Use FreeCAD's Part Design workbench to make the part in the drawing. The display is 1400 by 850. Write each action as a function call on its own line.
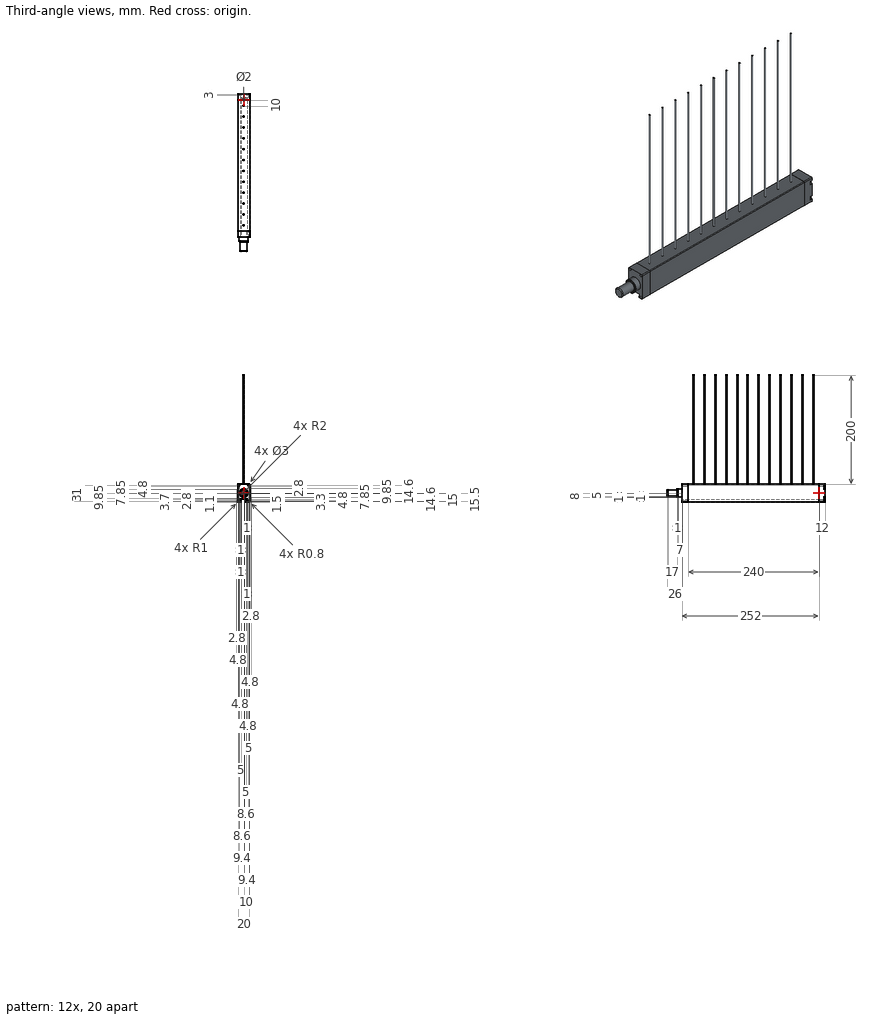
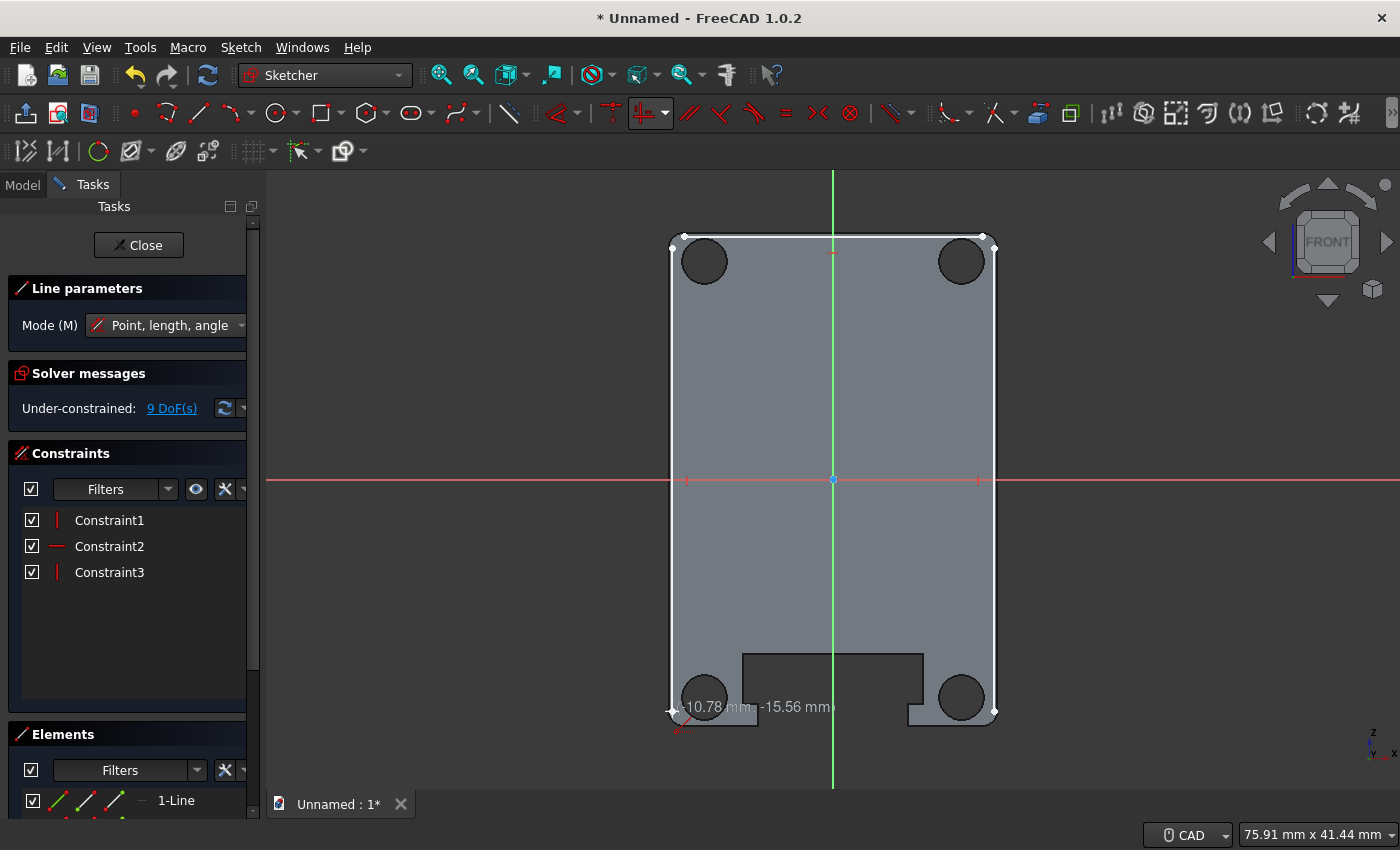
click(168, 114)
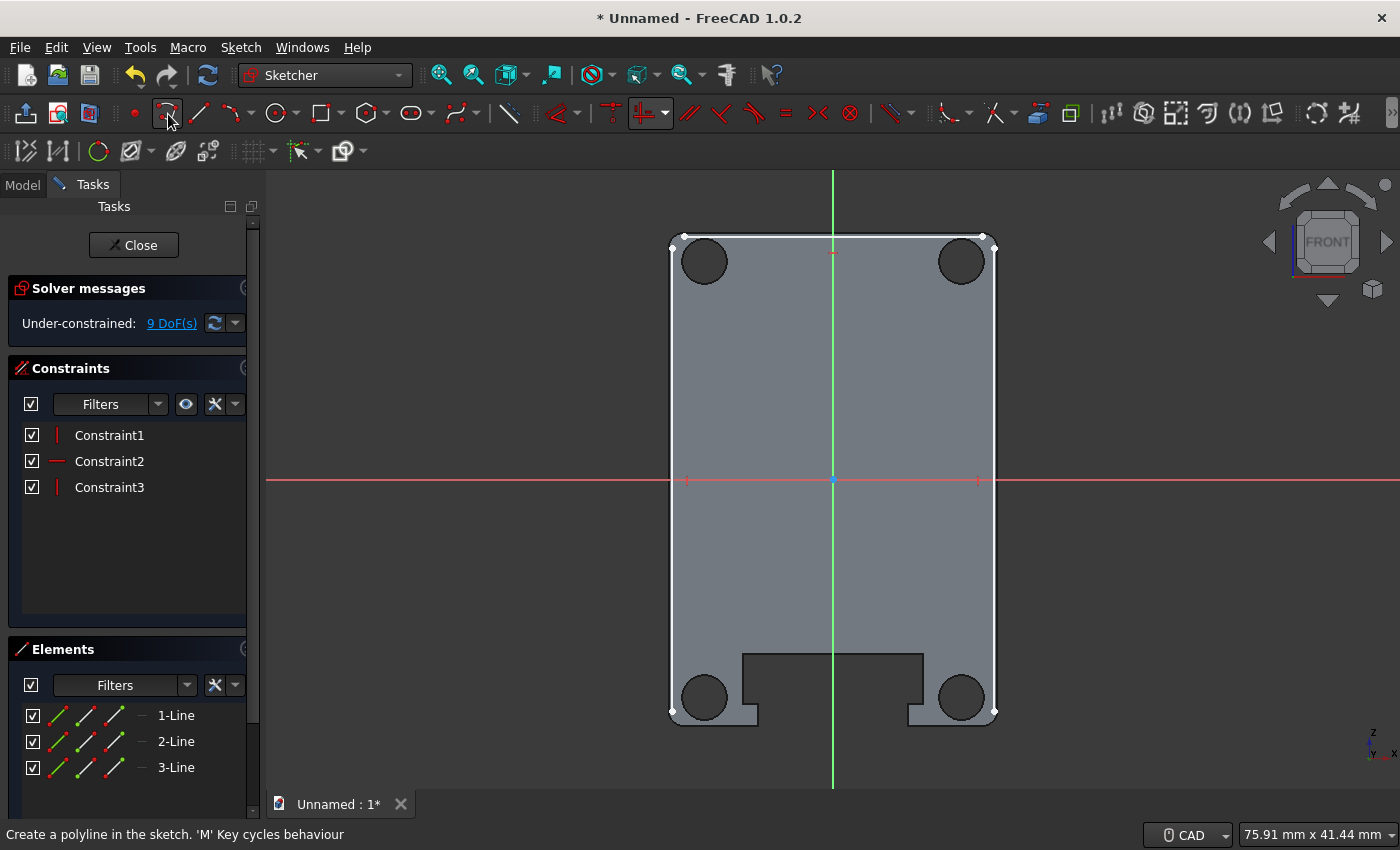
click(684, 723)
click(755, 723)
click(755, 707)
click(740, 707)
click(740, 651)
click(926, 651)
click(926, 707)
click(911, 707)
click(911, 723)
click(982, 723)
right_click(982, 723)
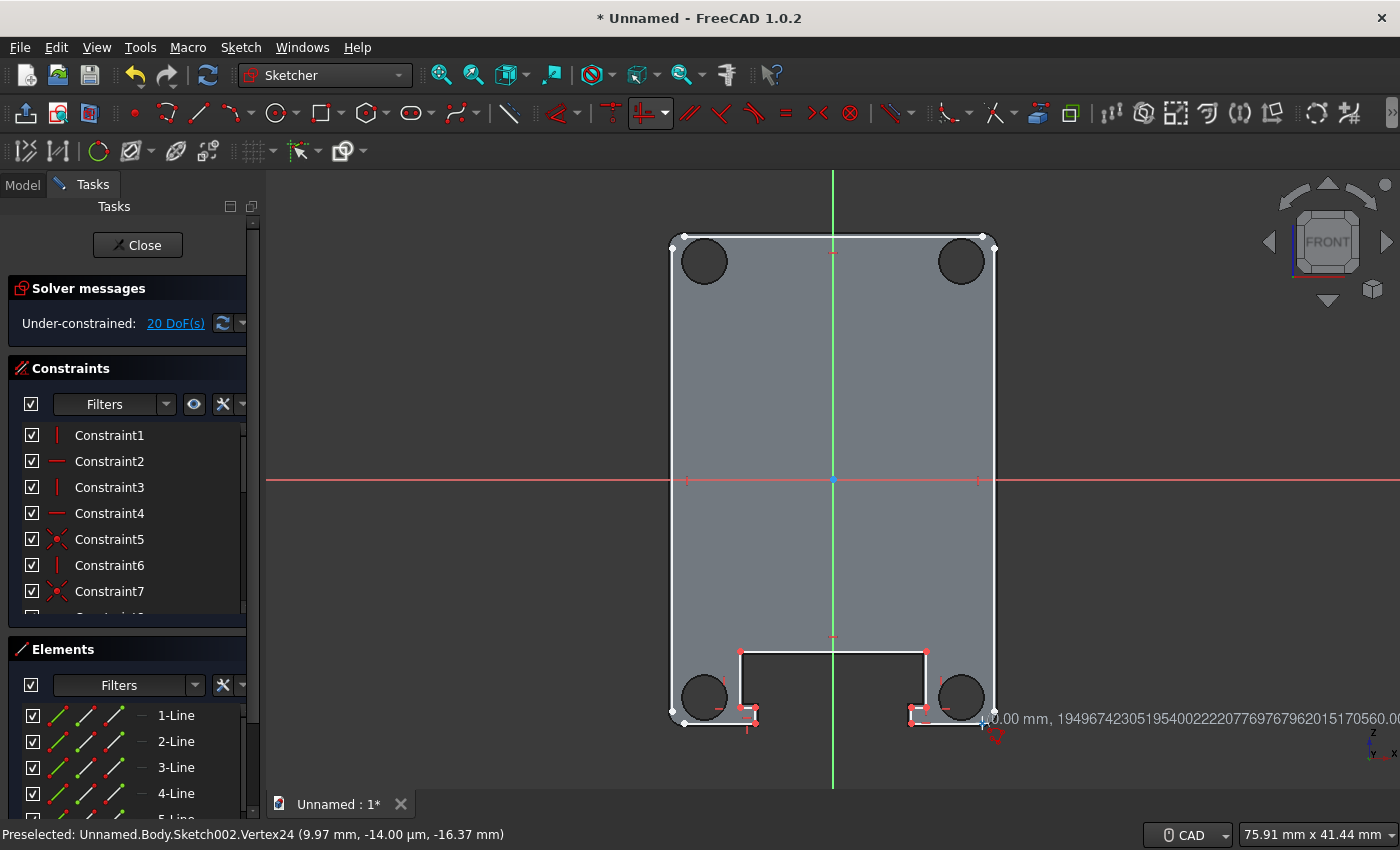
click(232, 114)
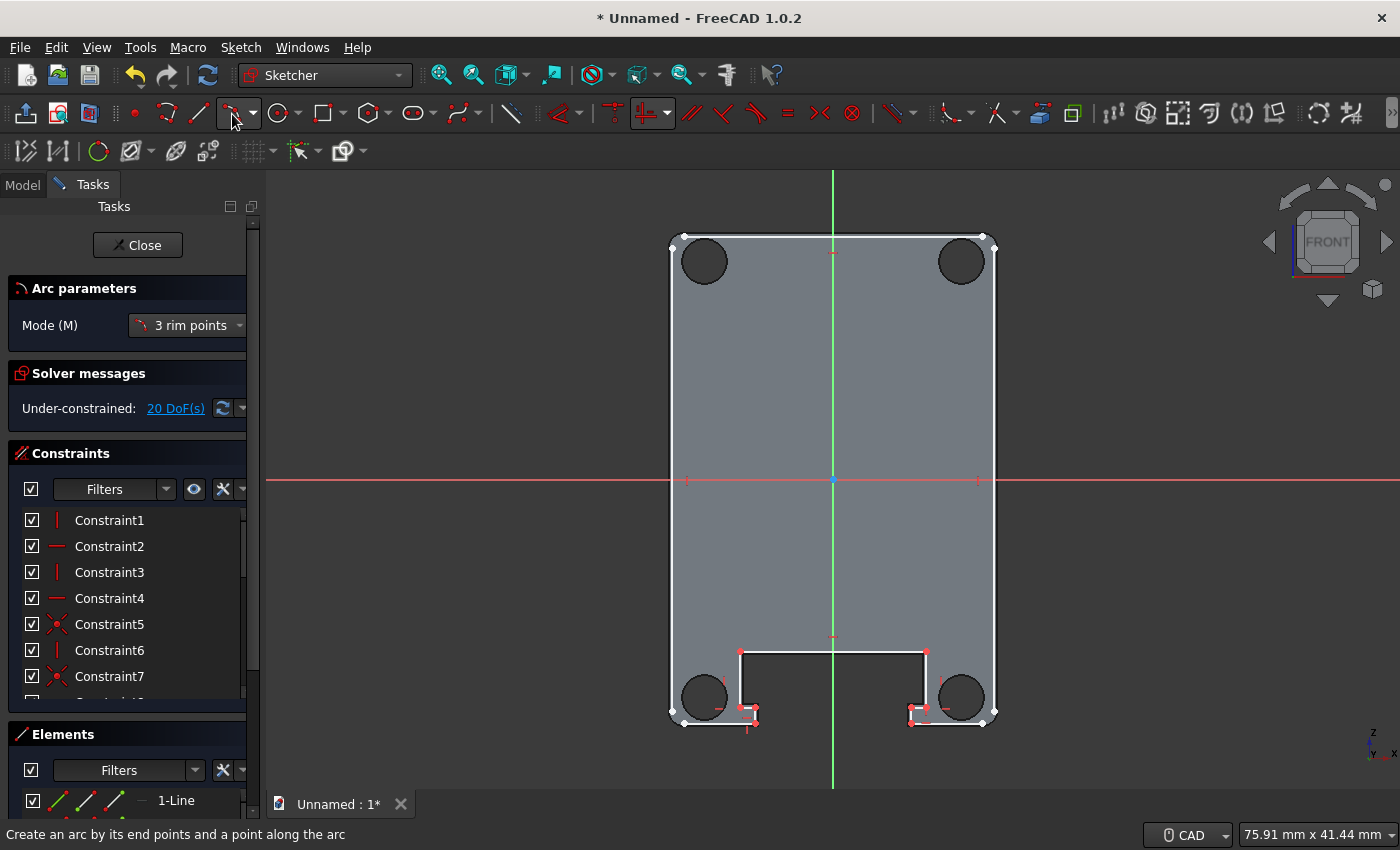
click(994, 249)
click(982, 237)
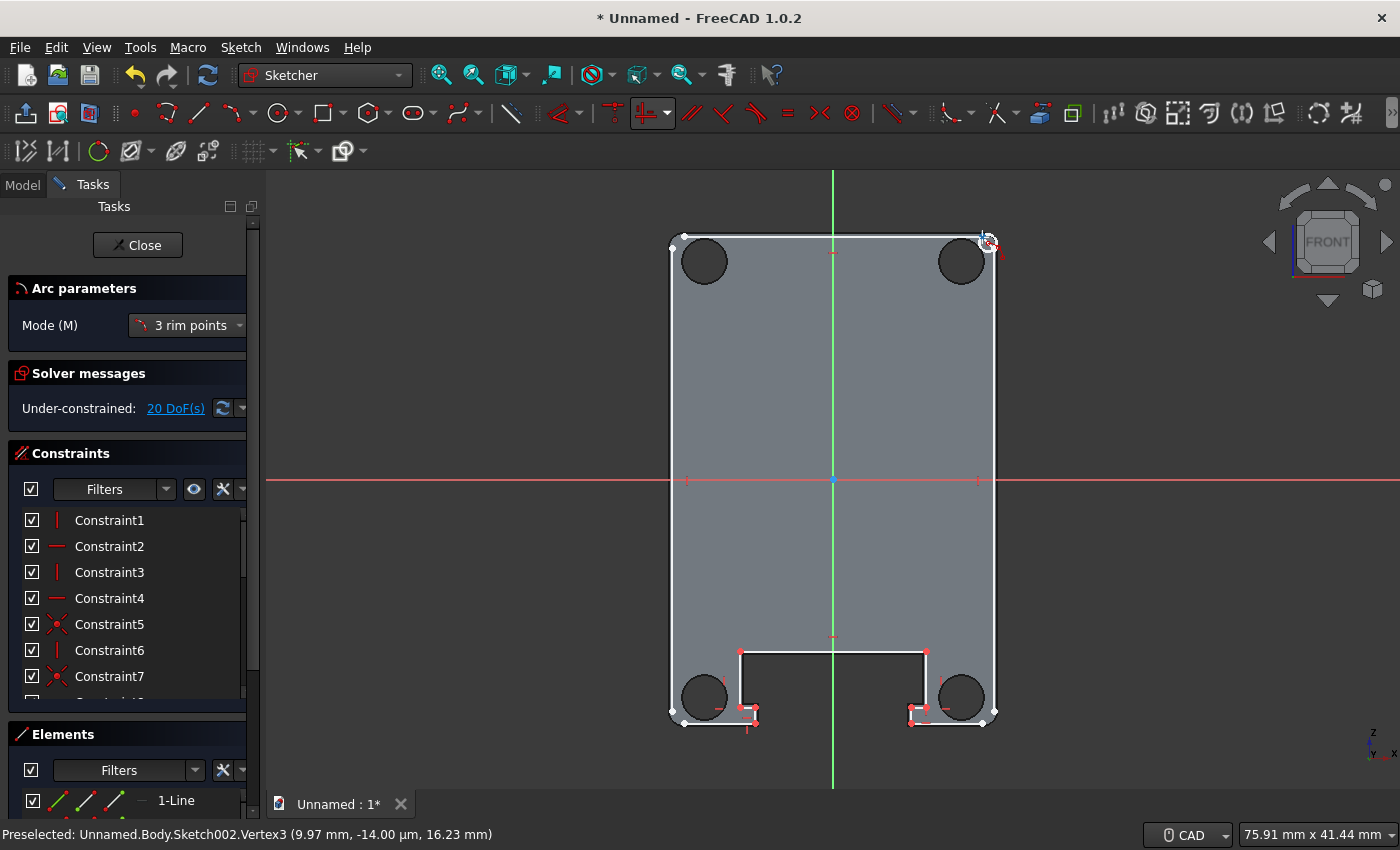
scroll(991, 240, up, 8)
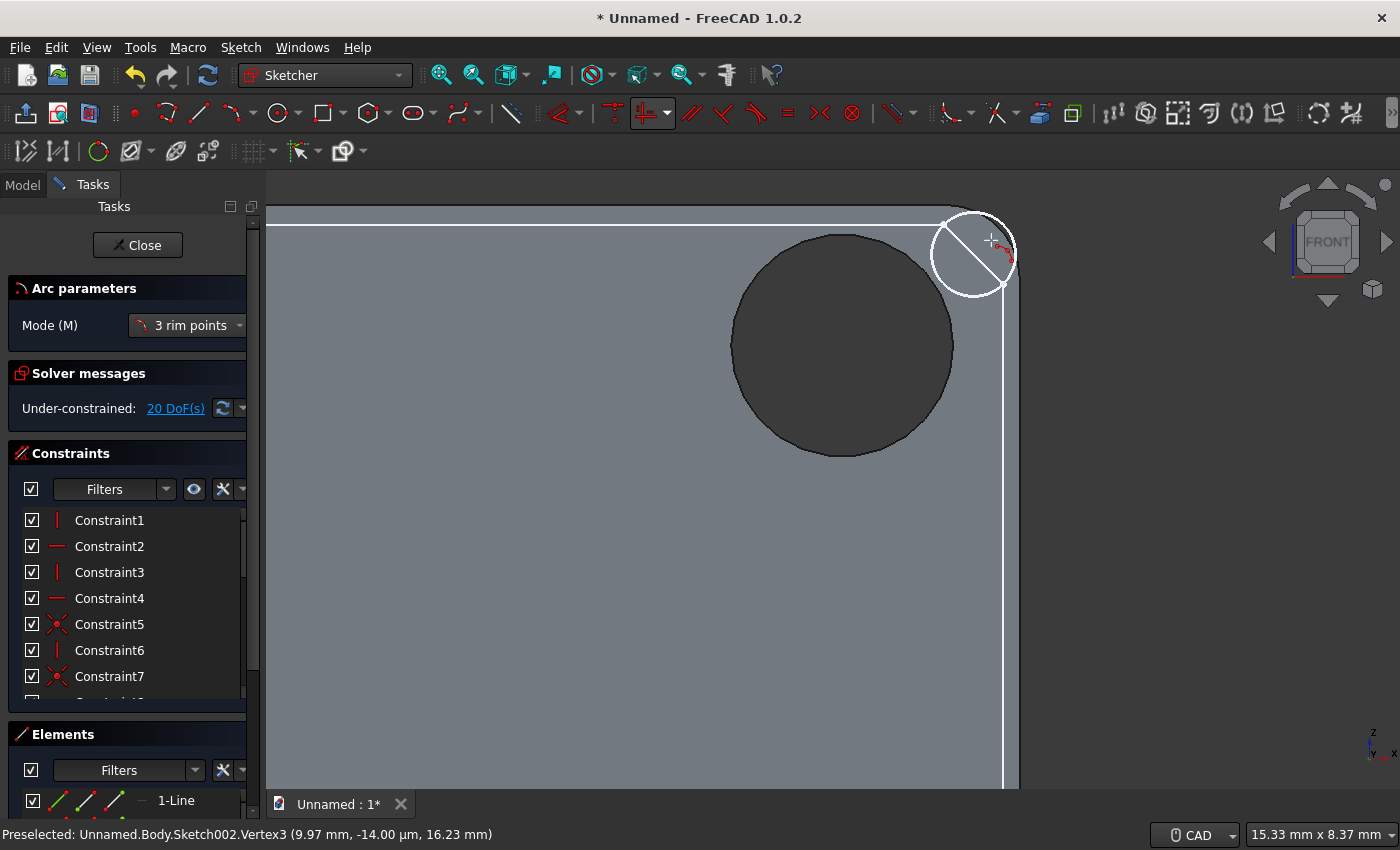
click(988, 237)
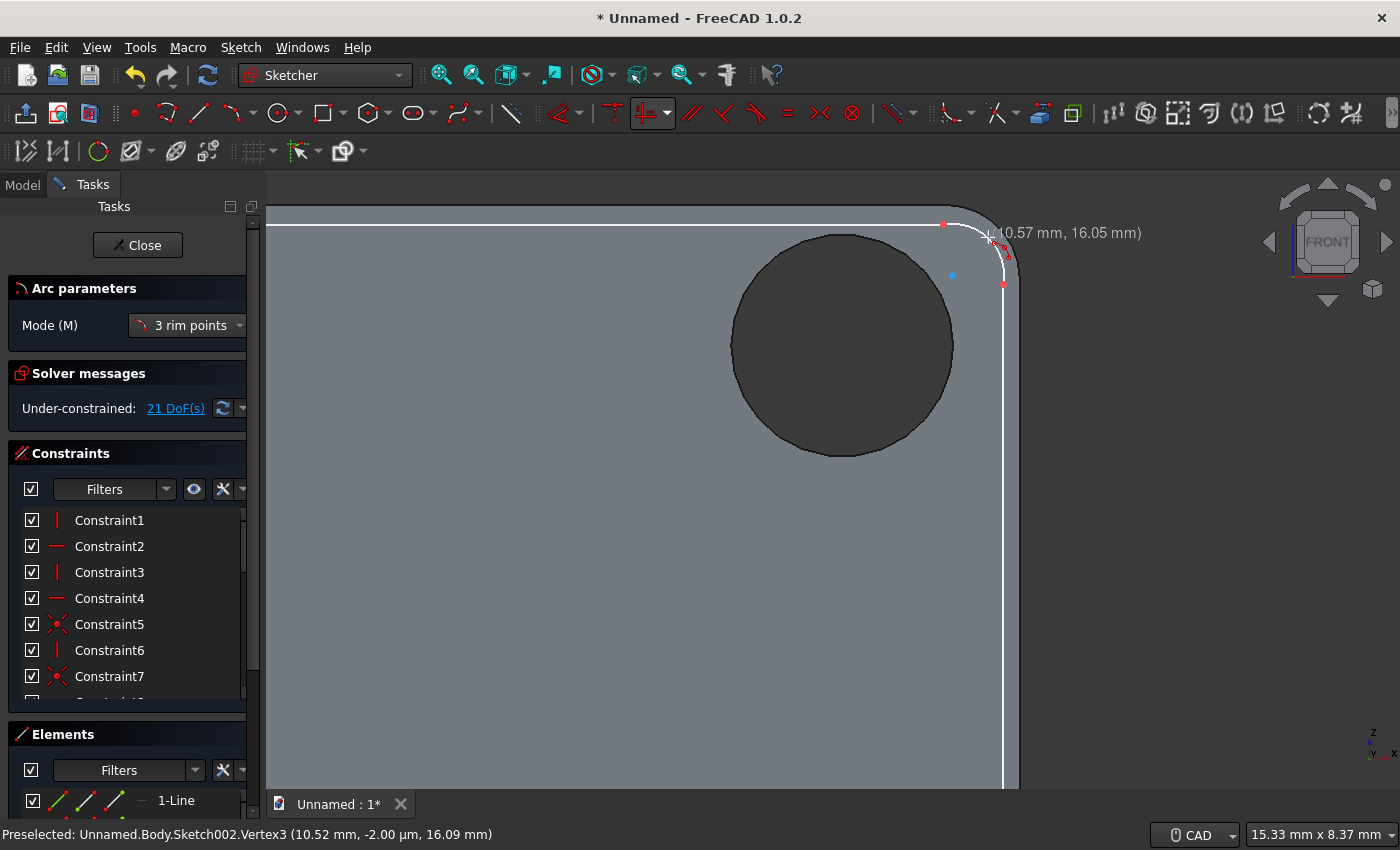
scroll(875, 292, down, 9)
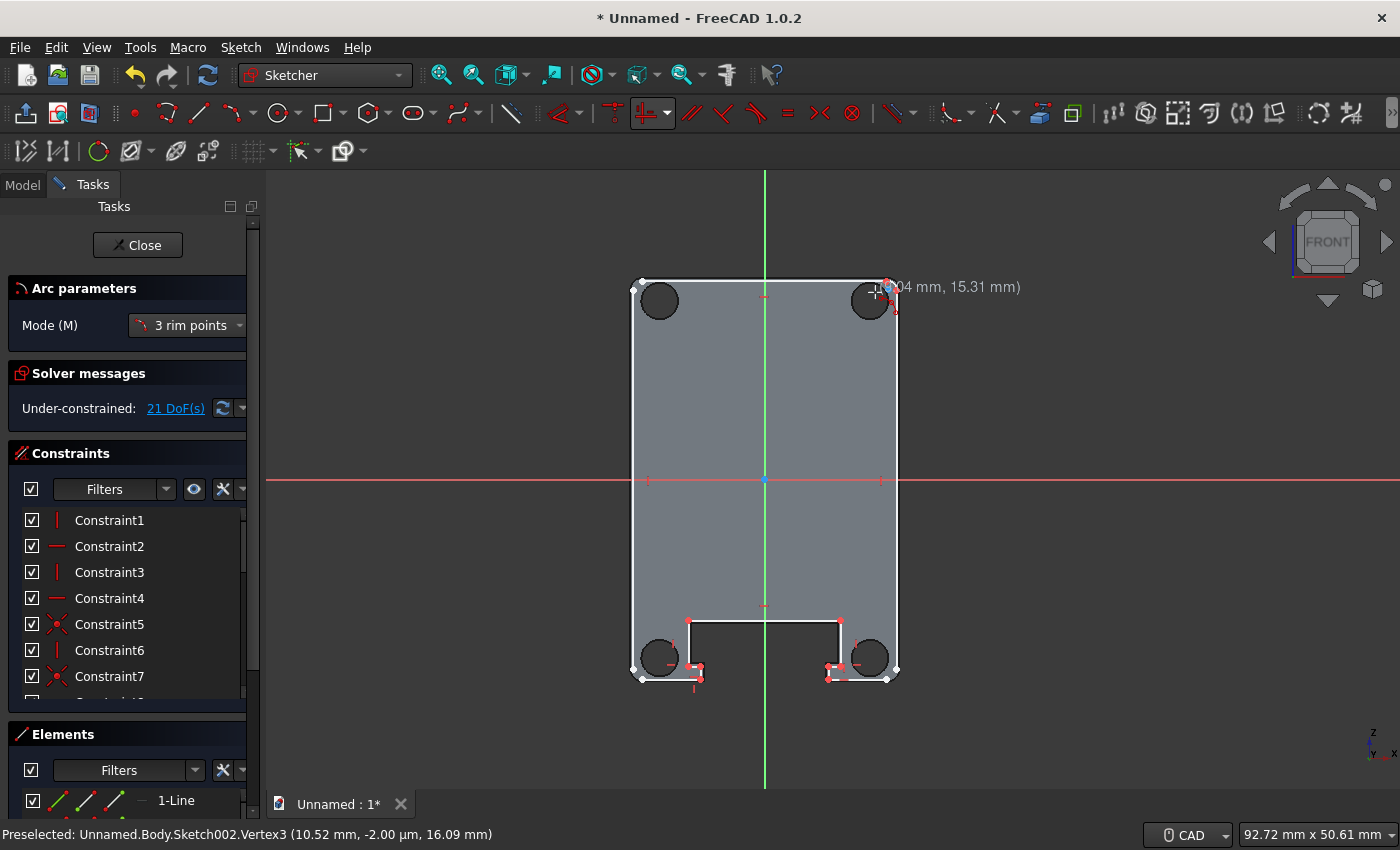
click(643, 281)
click(633, 291)